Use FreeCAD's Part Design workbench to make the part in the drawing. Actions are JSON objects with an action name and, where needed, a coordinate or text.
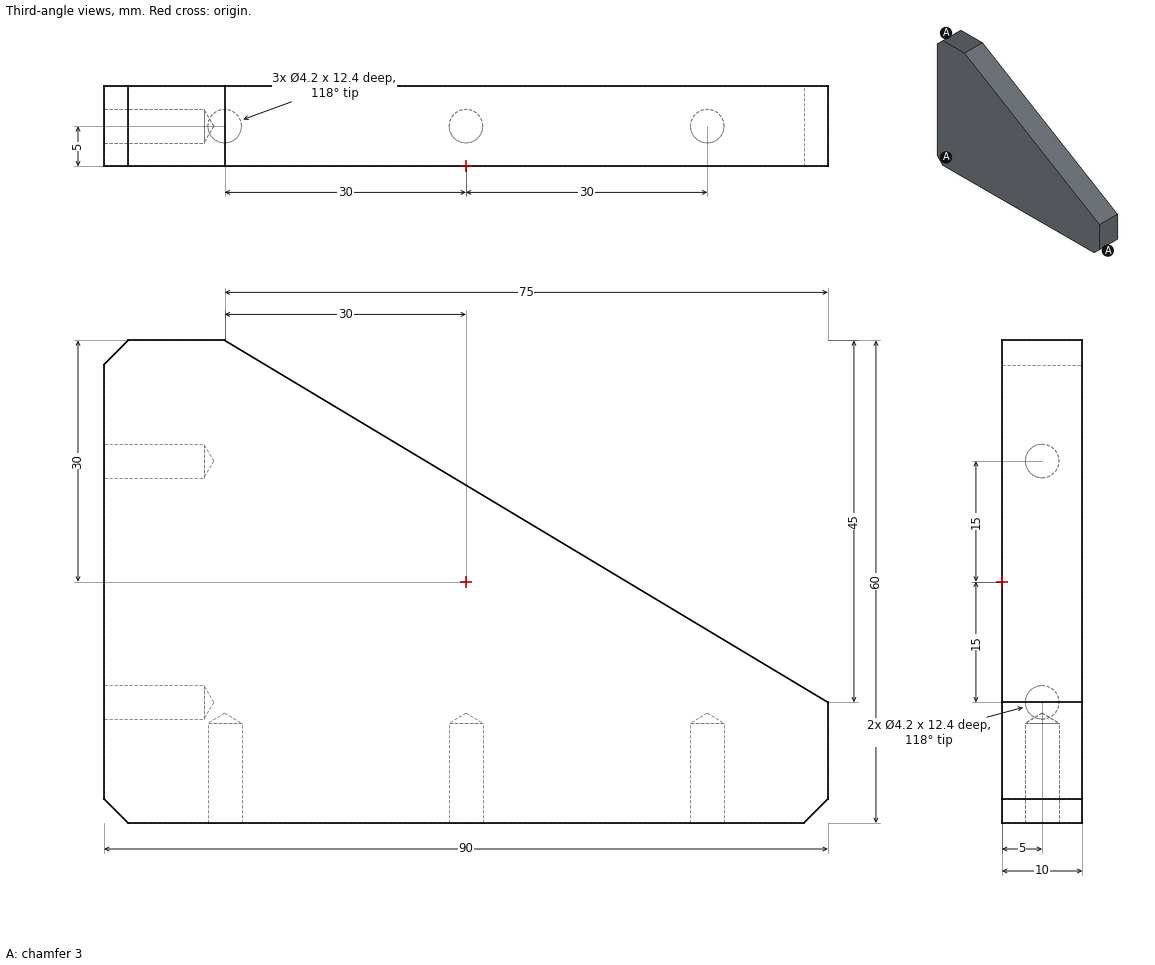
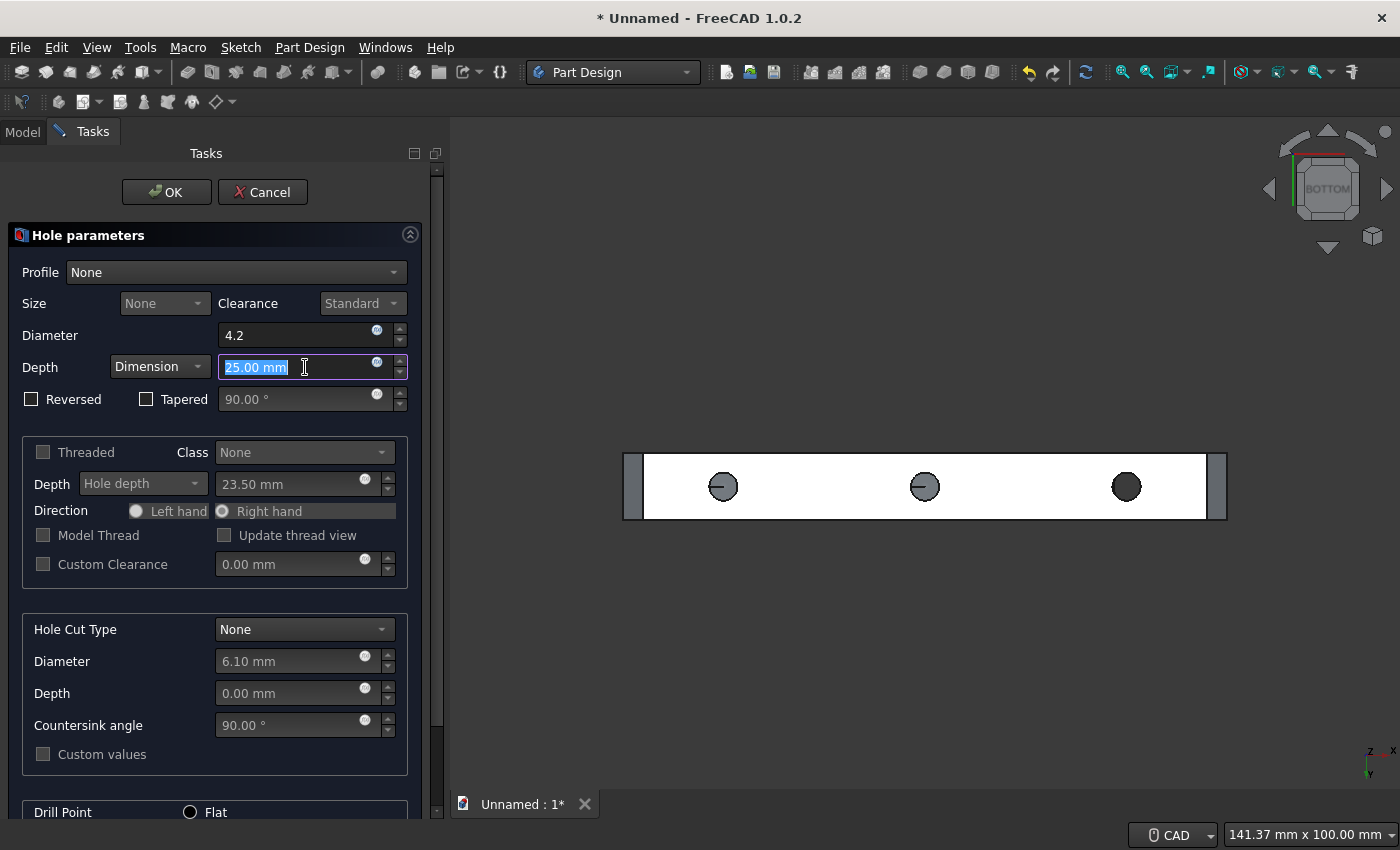
{"action": "type", "text": "12.4"}
{"action": "key", "text": "Tab"}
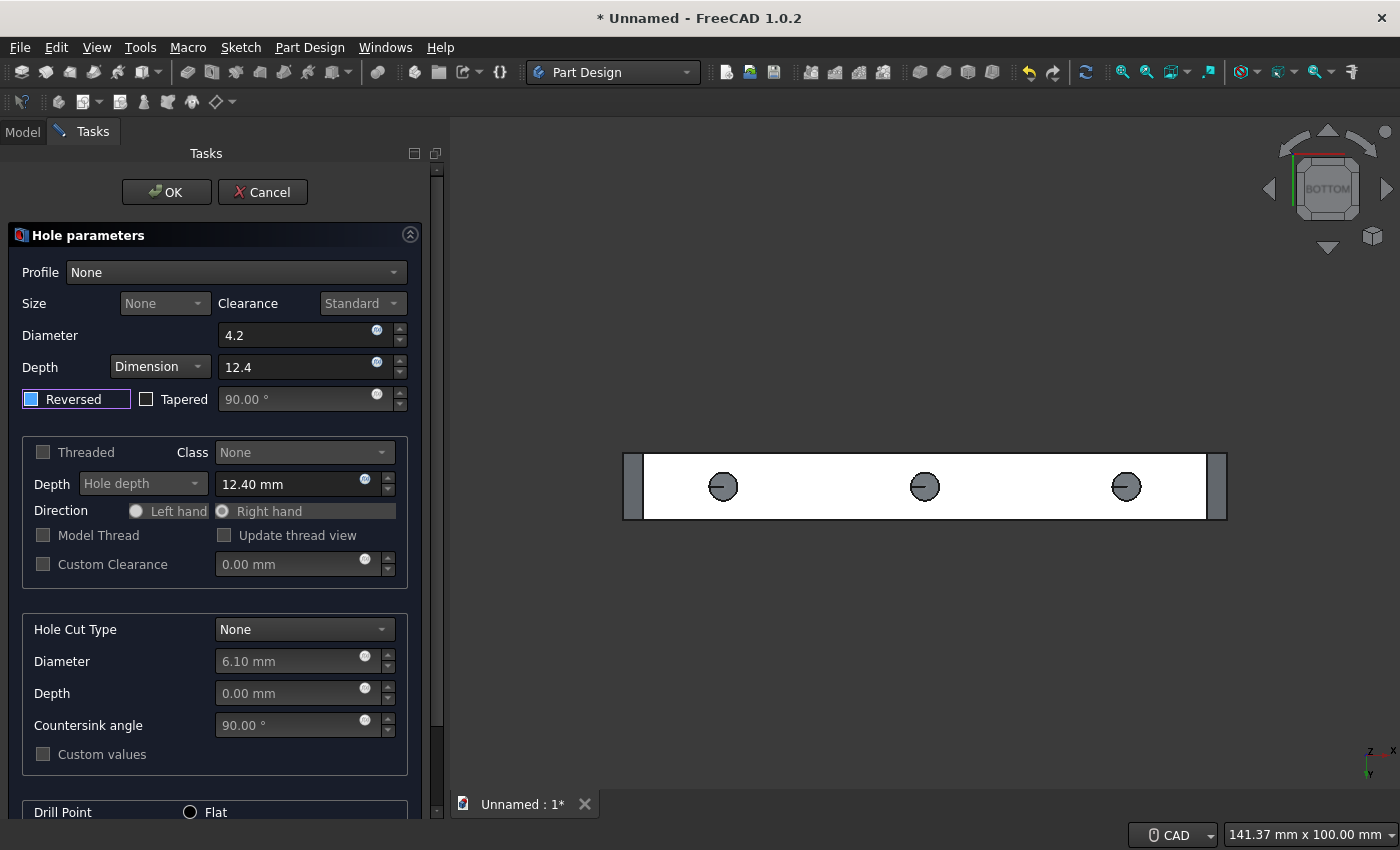
{"action": "left_click", "coordinate": [167, 192]}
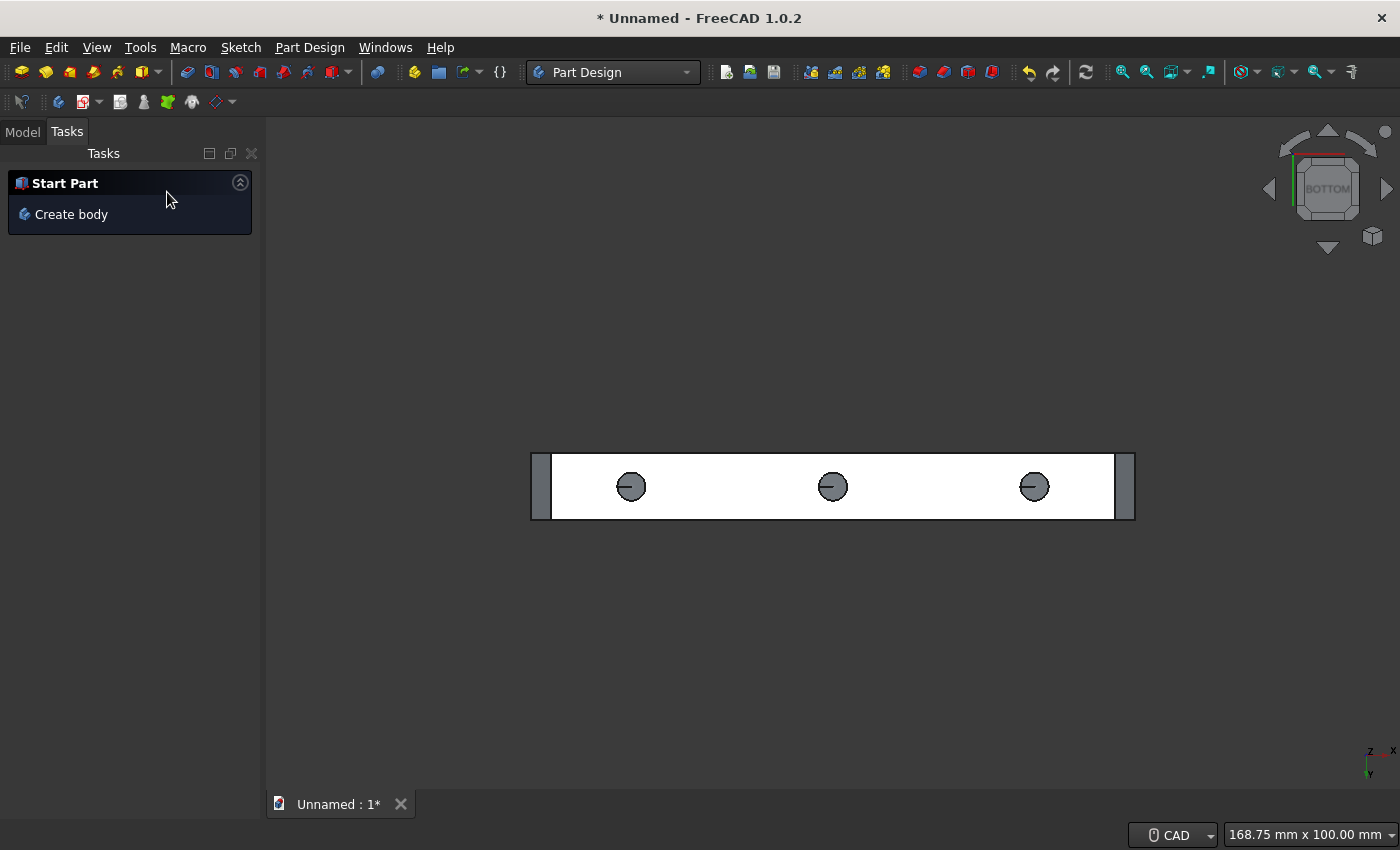
{"action": "key", "text": "0"}